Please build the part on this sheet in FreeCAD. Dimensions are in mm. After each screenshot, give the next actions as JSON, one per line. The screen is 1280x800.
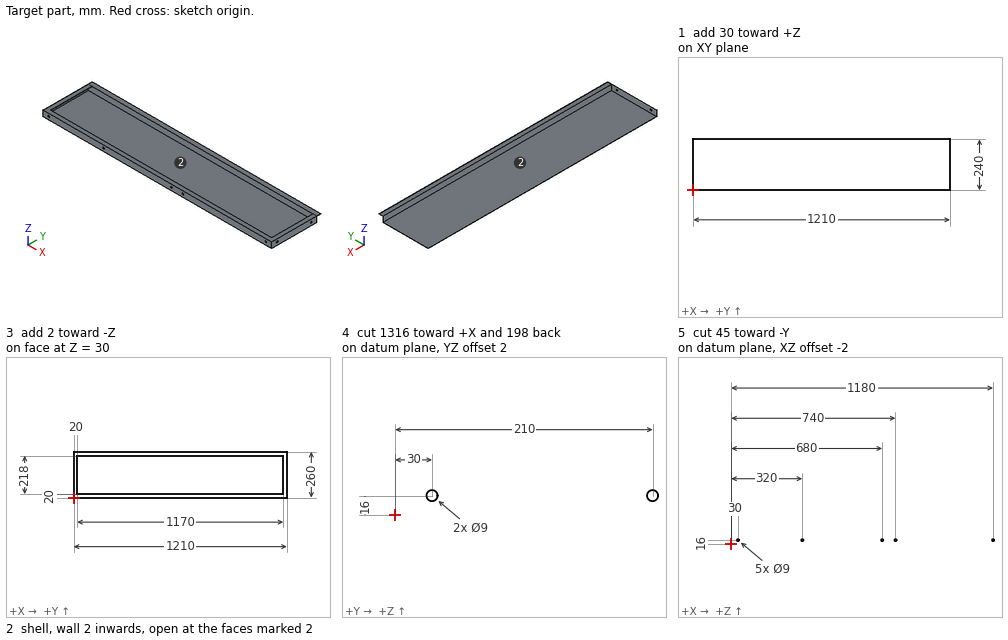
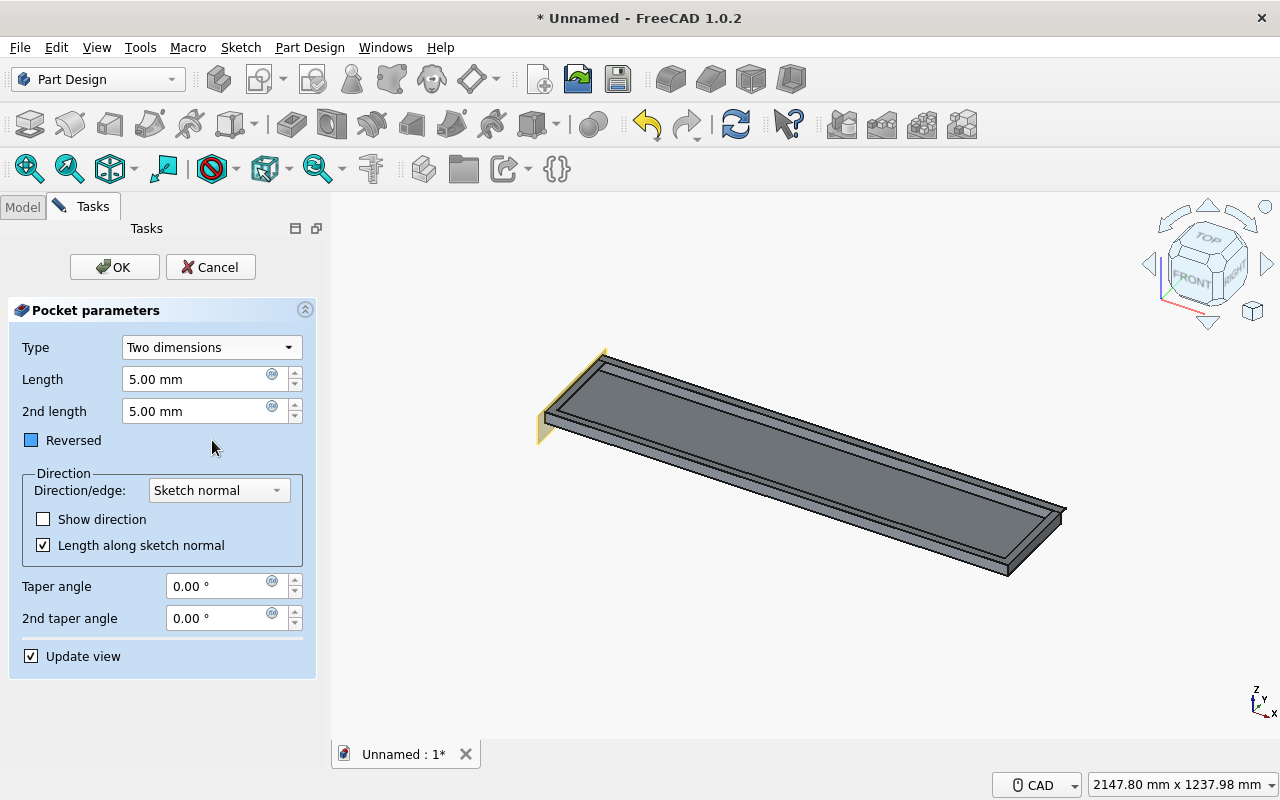
{"action": "triple_click", "coordinate": [204, 379]}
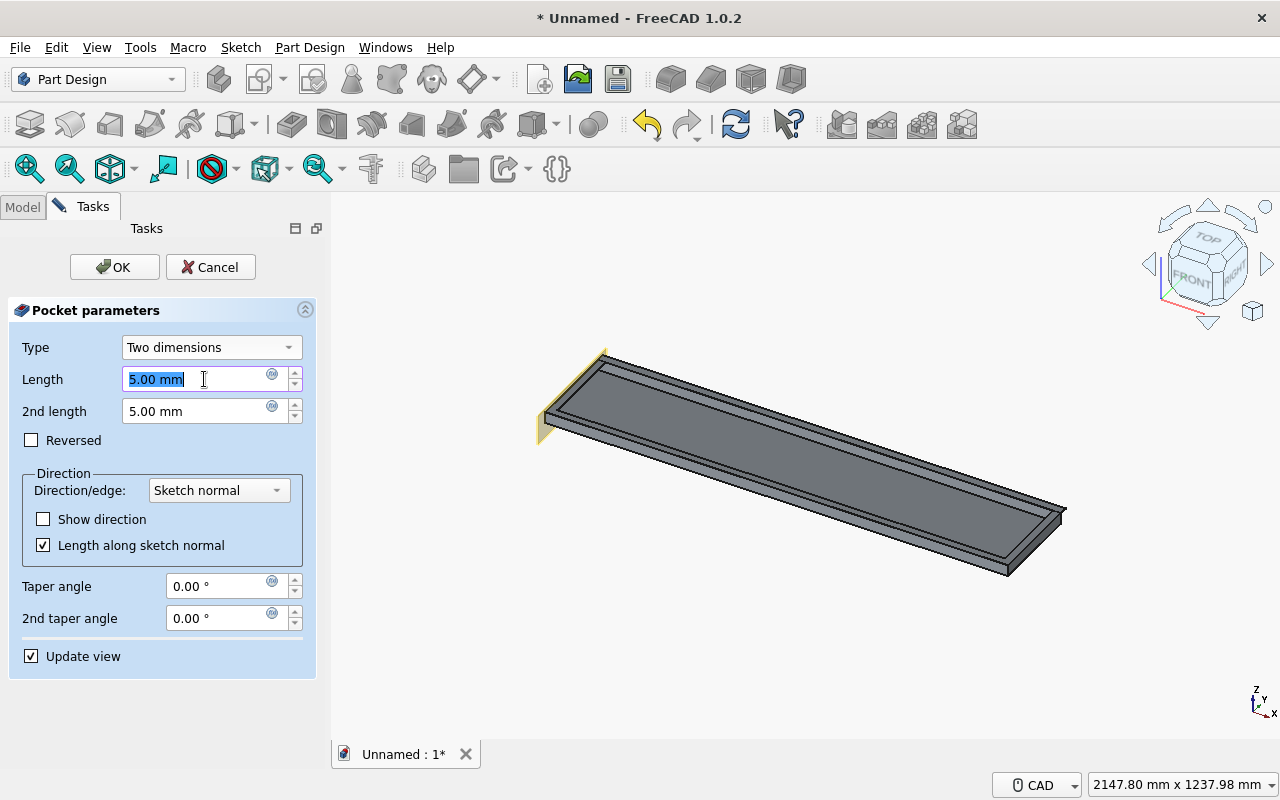
{"action": "type", "text": "1316"}
{"action": "key", "text": "Tab"}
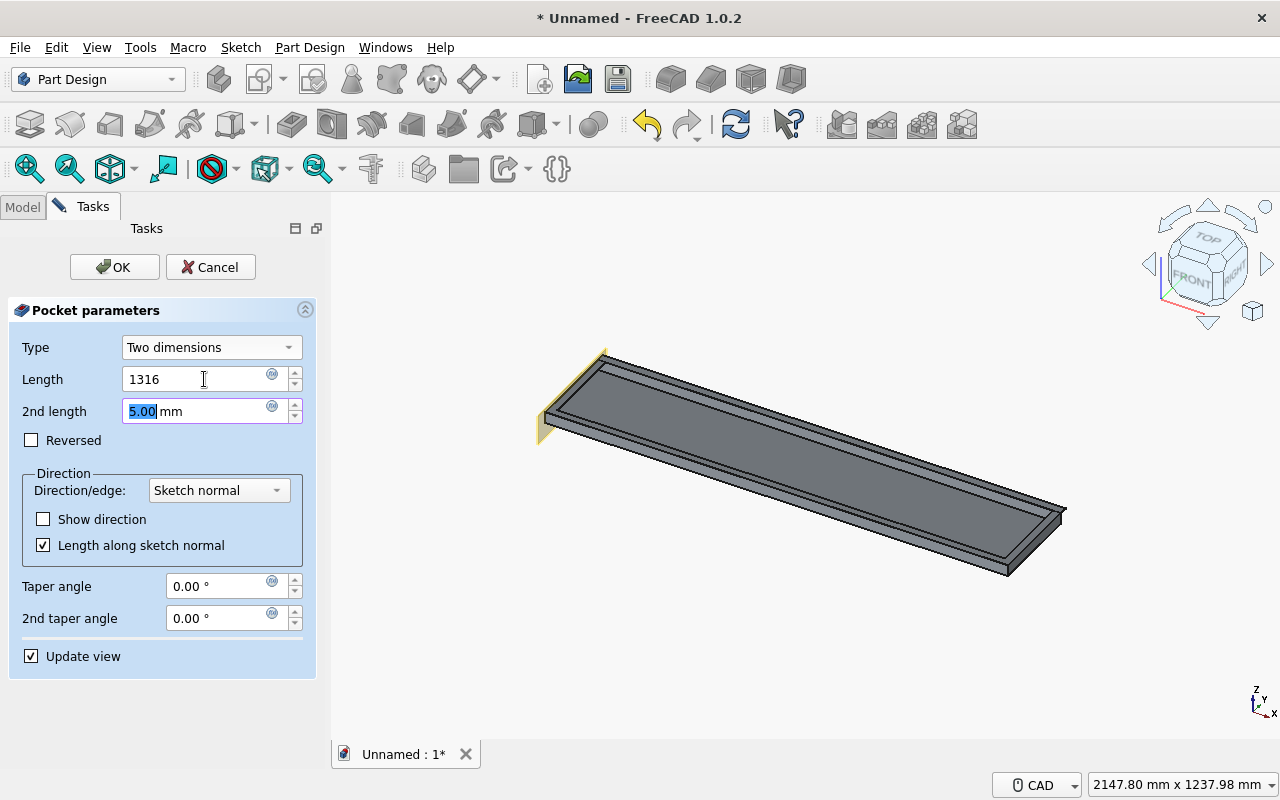
{"action": "type", "text": "198"}
{"action": "key", "text": "Tab"}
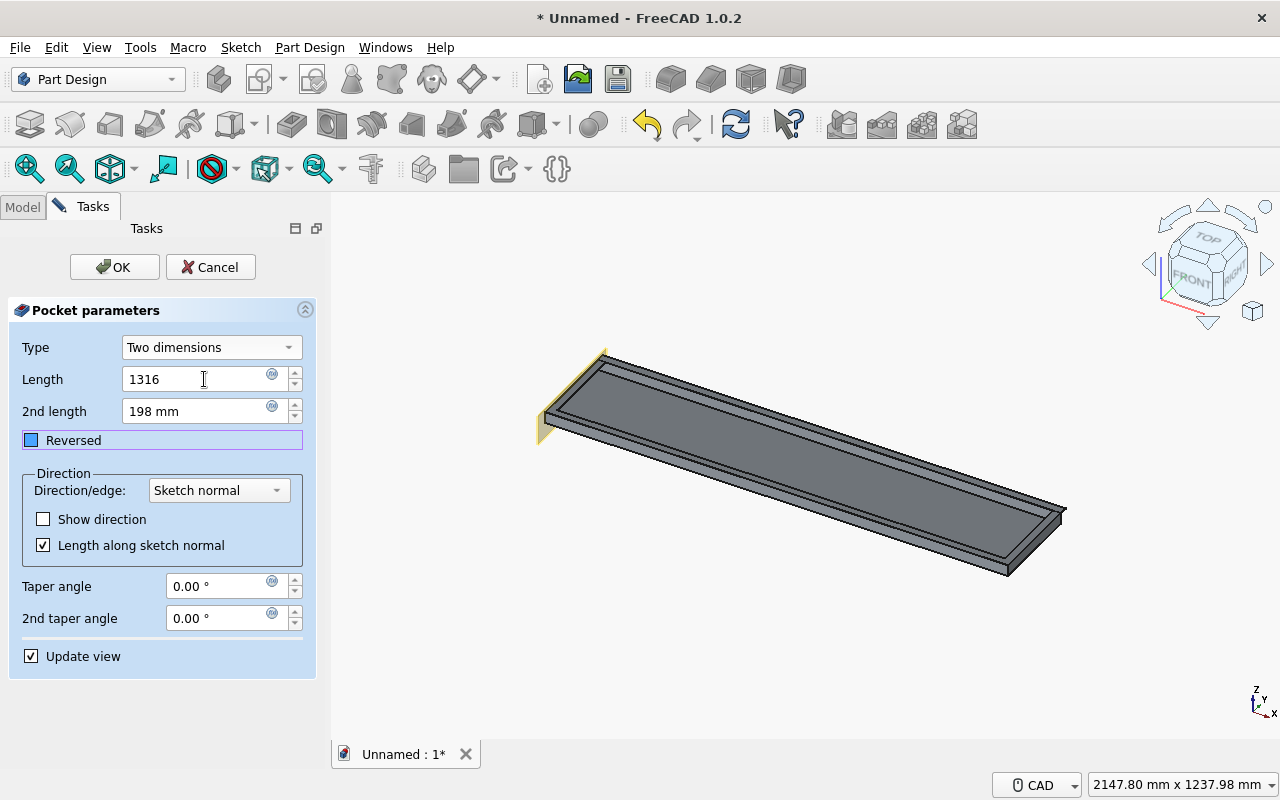
{"action": "left_click", "coordinate": [30, 440]}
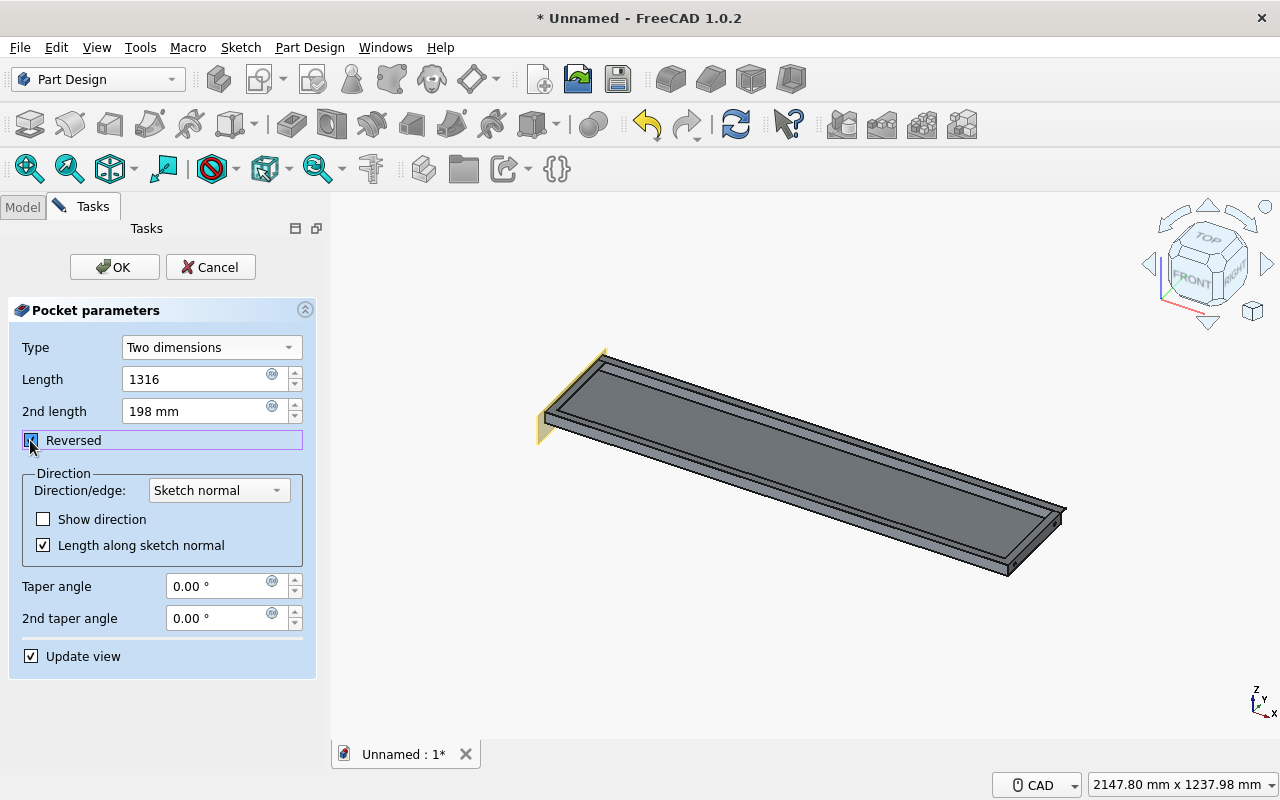
{"action": "left_click", "coordinate": [115, 267]}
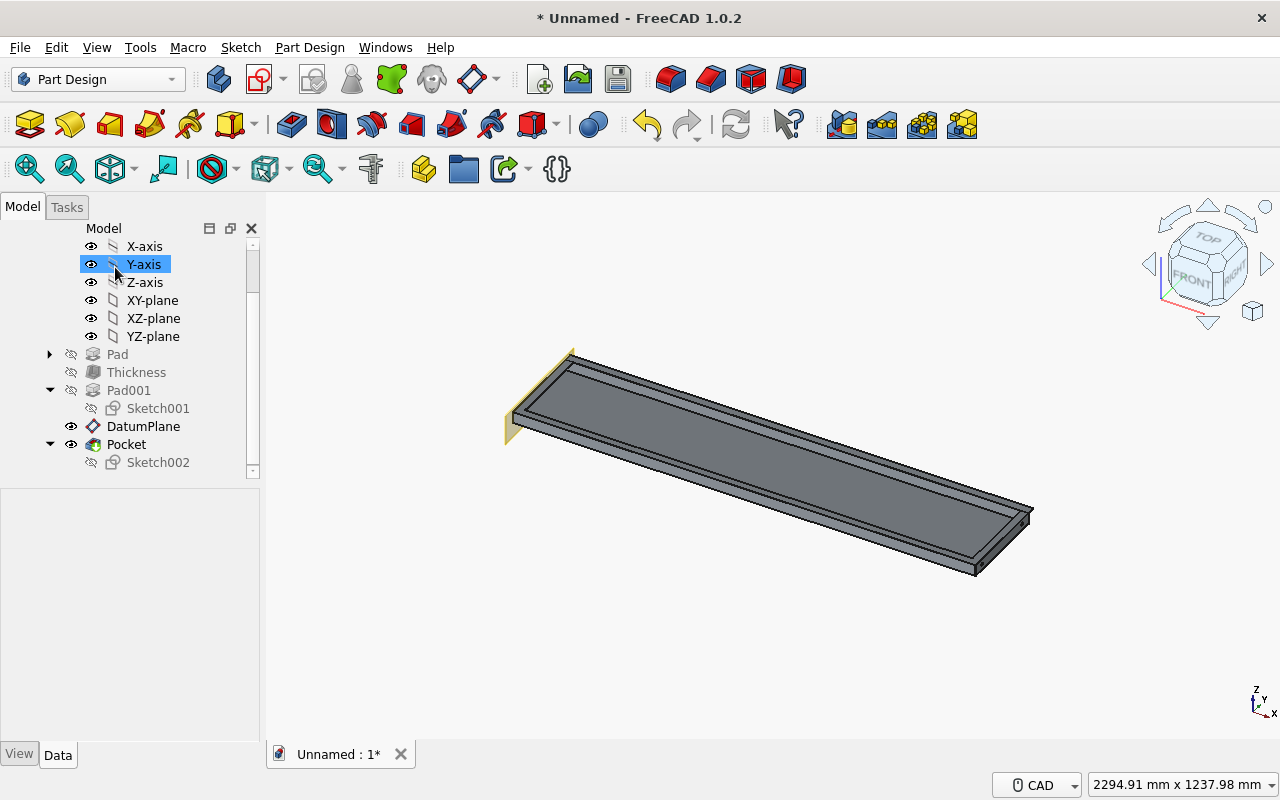
{"action": "left_click", "coordinate": [116, 426]}
{"action": "key", "text": "space"}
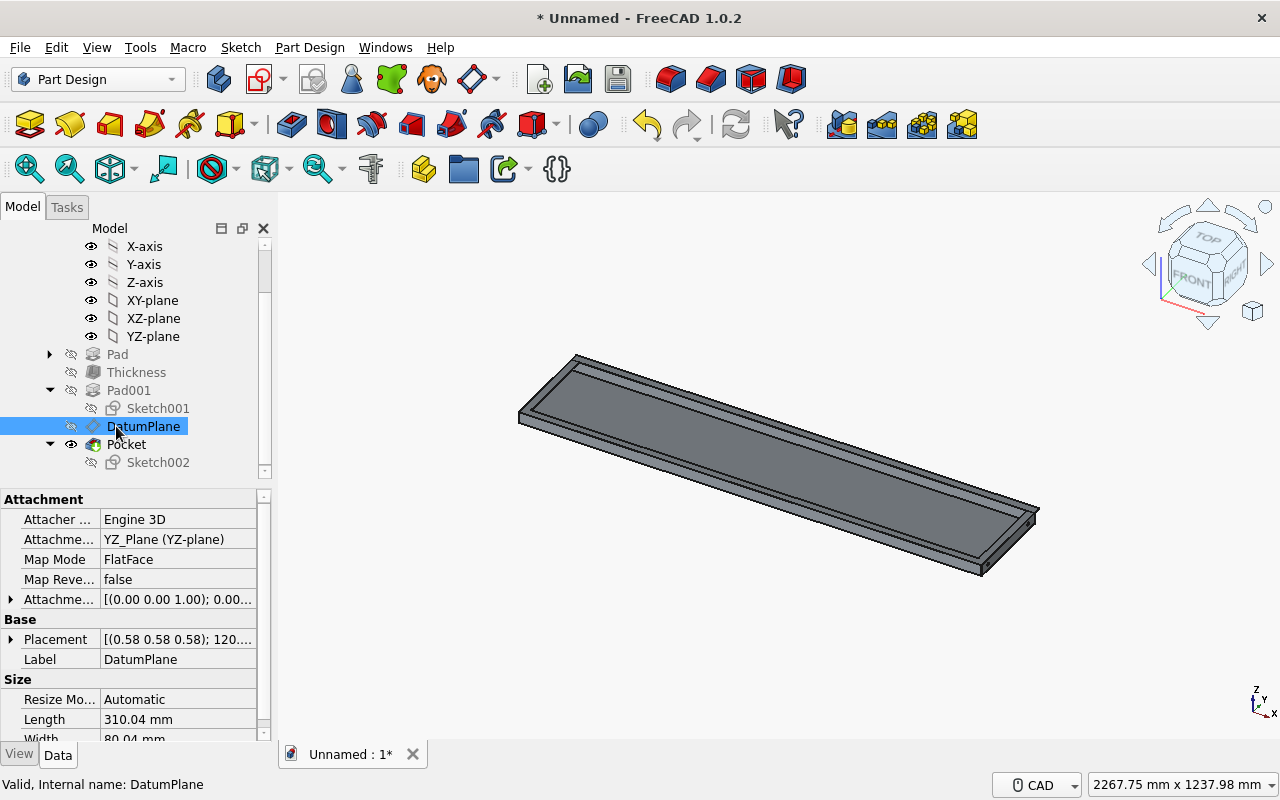
{"action": "scroll", "coordinate": [160, 350], "scroll_direction": "down", "scroll_amount": 3}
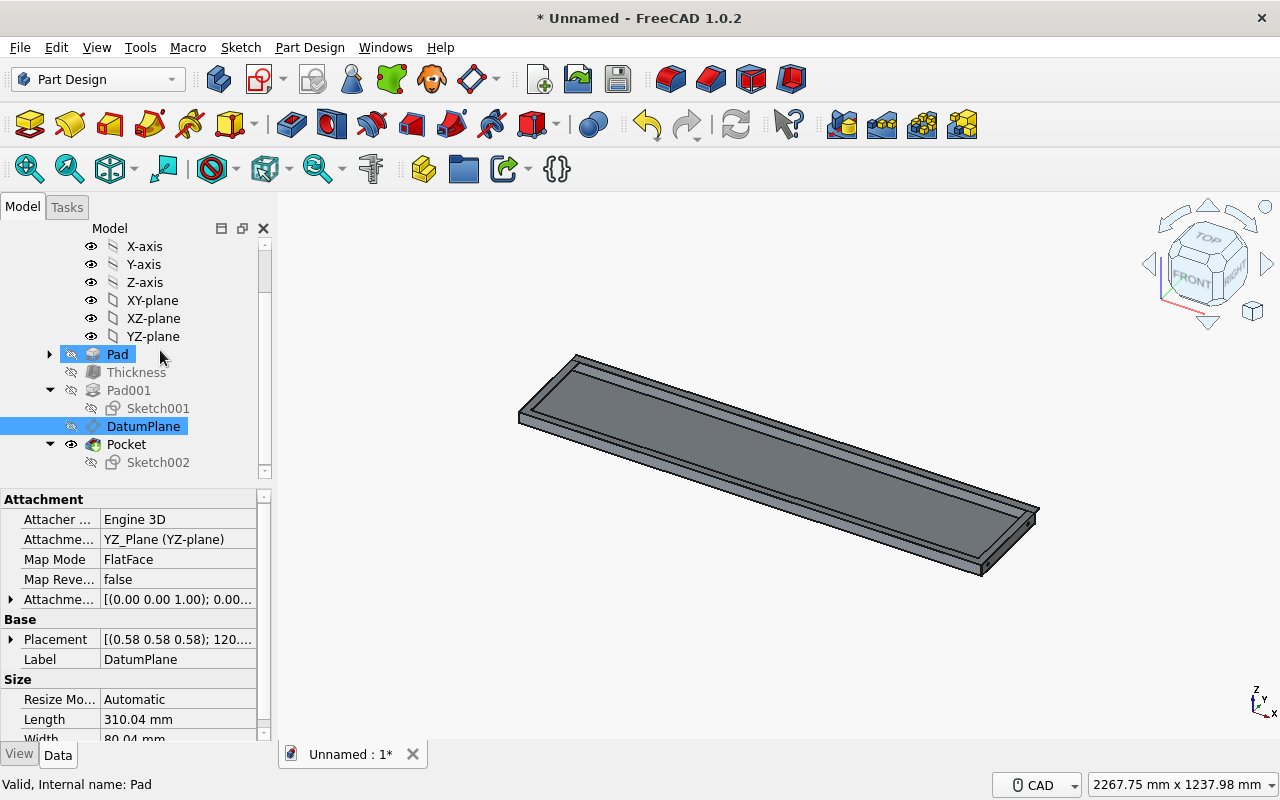
{"action": "scroll", "coordinate": [160, 350], "scroll_direction": "up", "scroll_amount": 15}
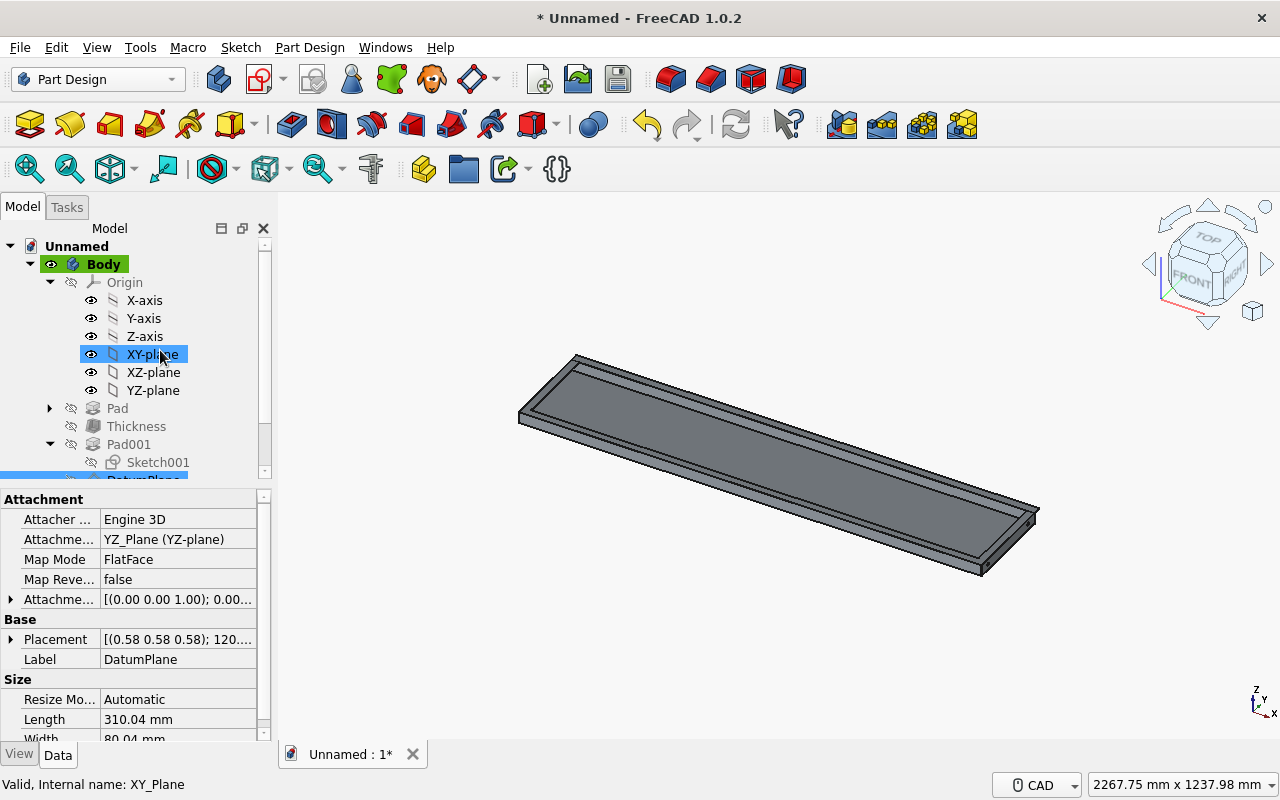
{"action": "left_click", "coordinate": [136, 372]}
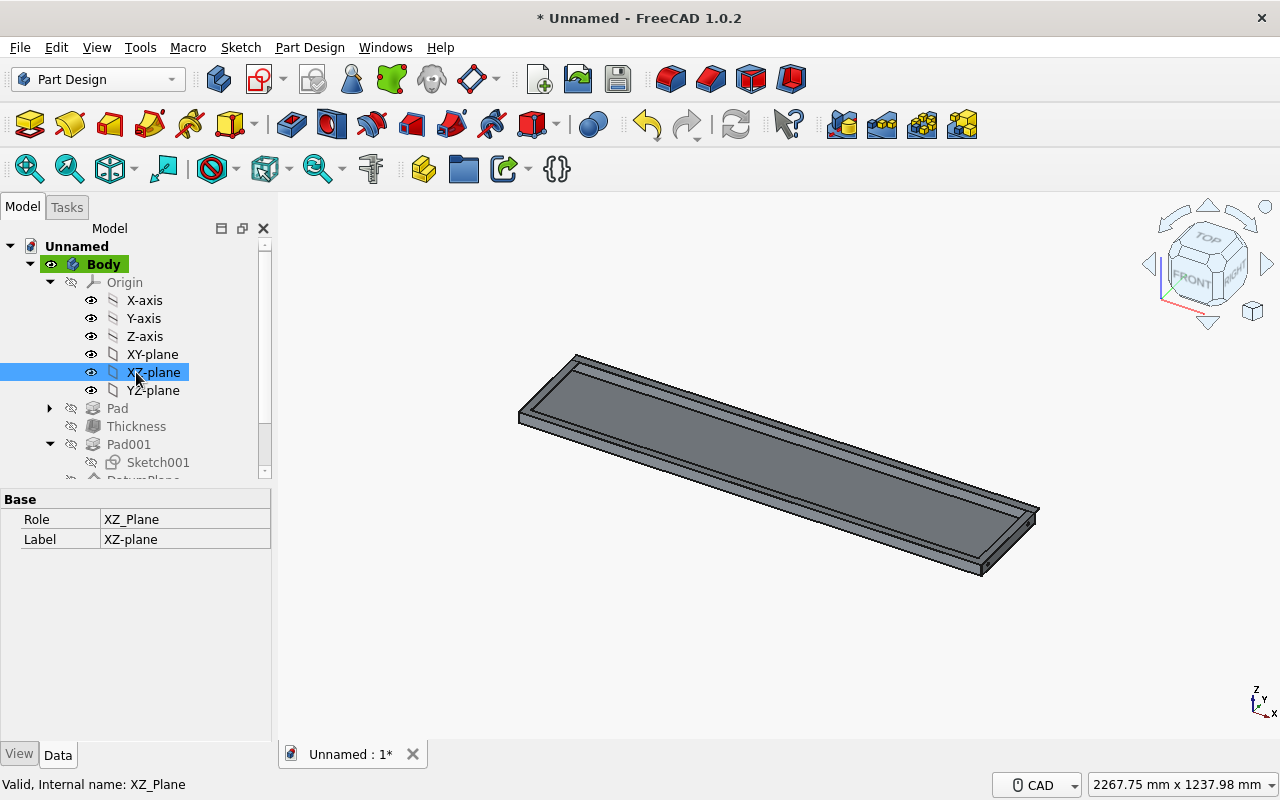
{"action": "left_click", "coordinate": [472, 80]}